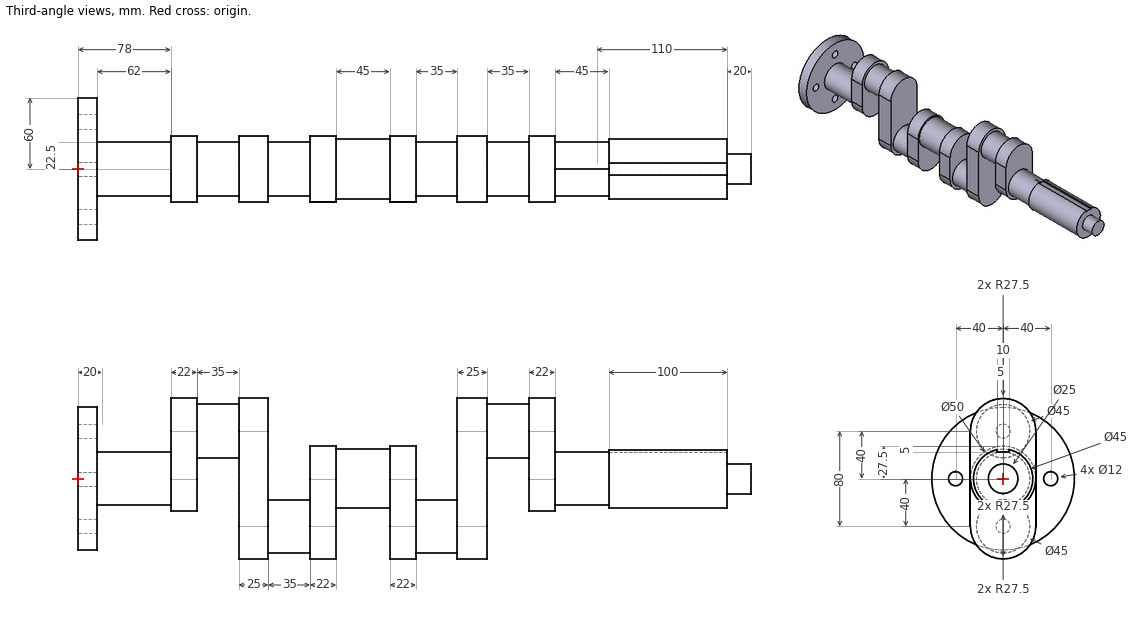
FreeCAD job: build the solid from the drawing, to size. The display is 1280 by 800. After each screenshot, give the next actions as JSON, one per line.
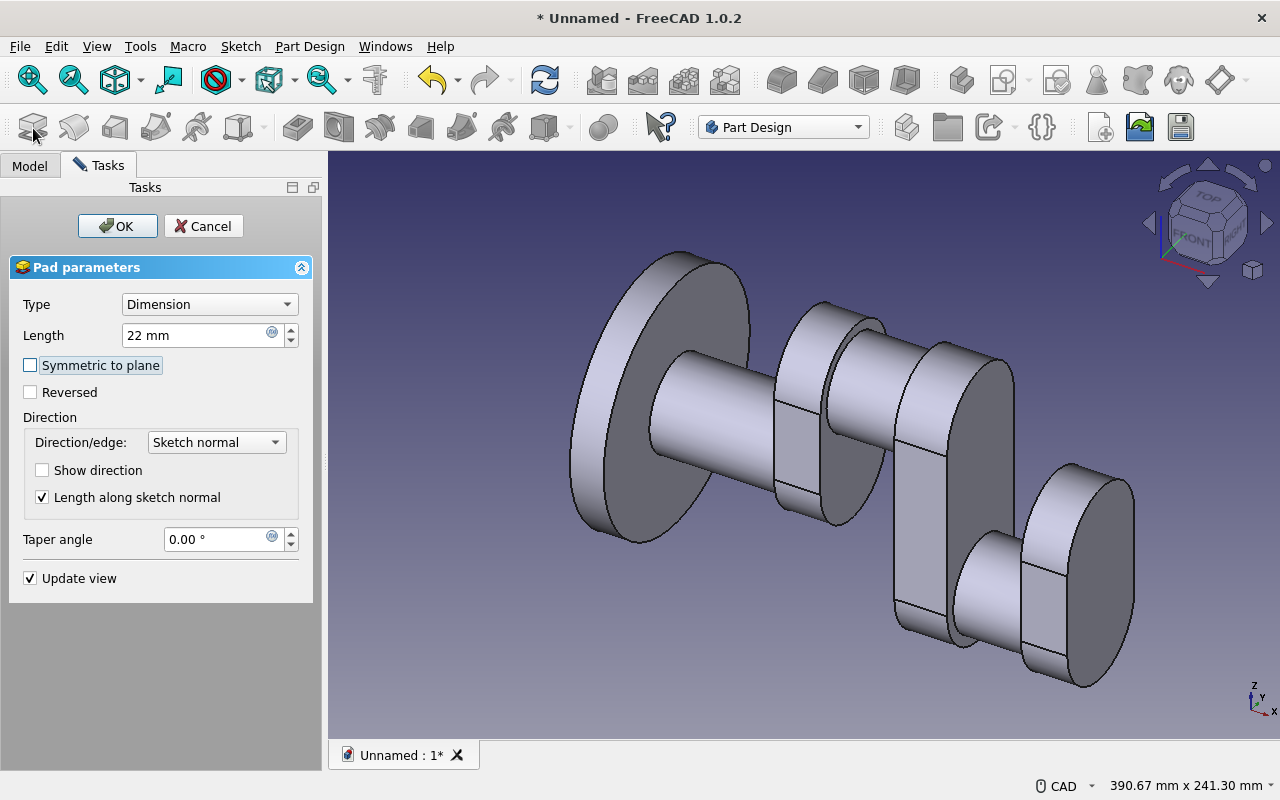
{"action": "left_click", "coordinate": [118, 226]}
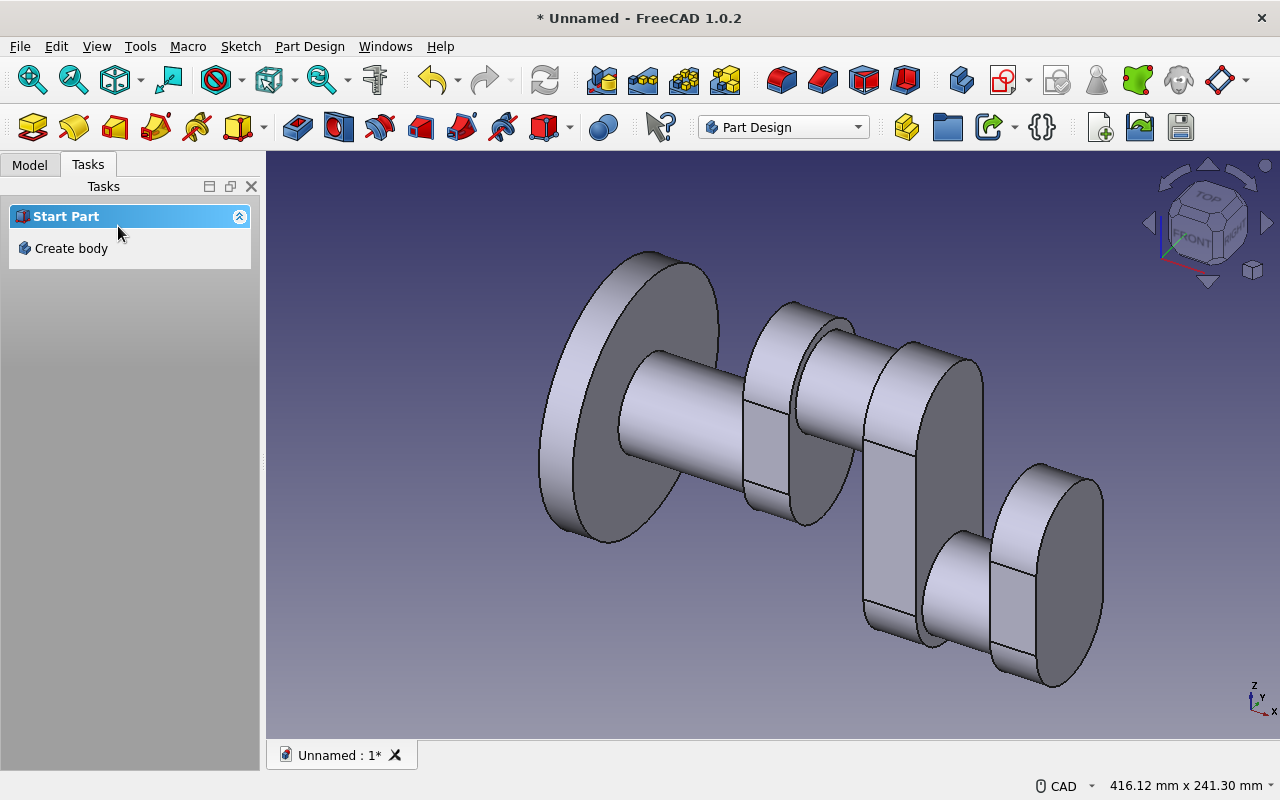
{"action": "left_click", "coordinate": [33, 80]}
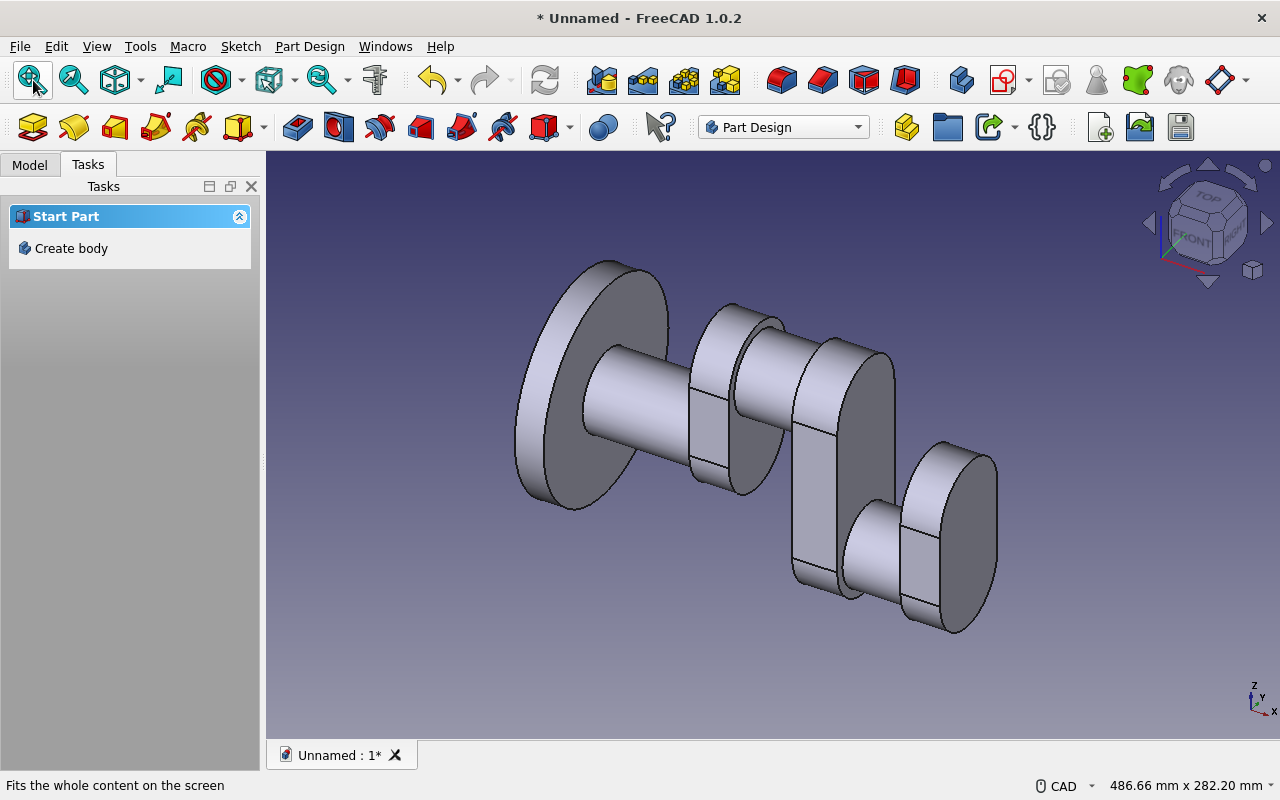
{"action": "left_click", "coordinate": [969, 520]}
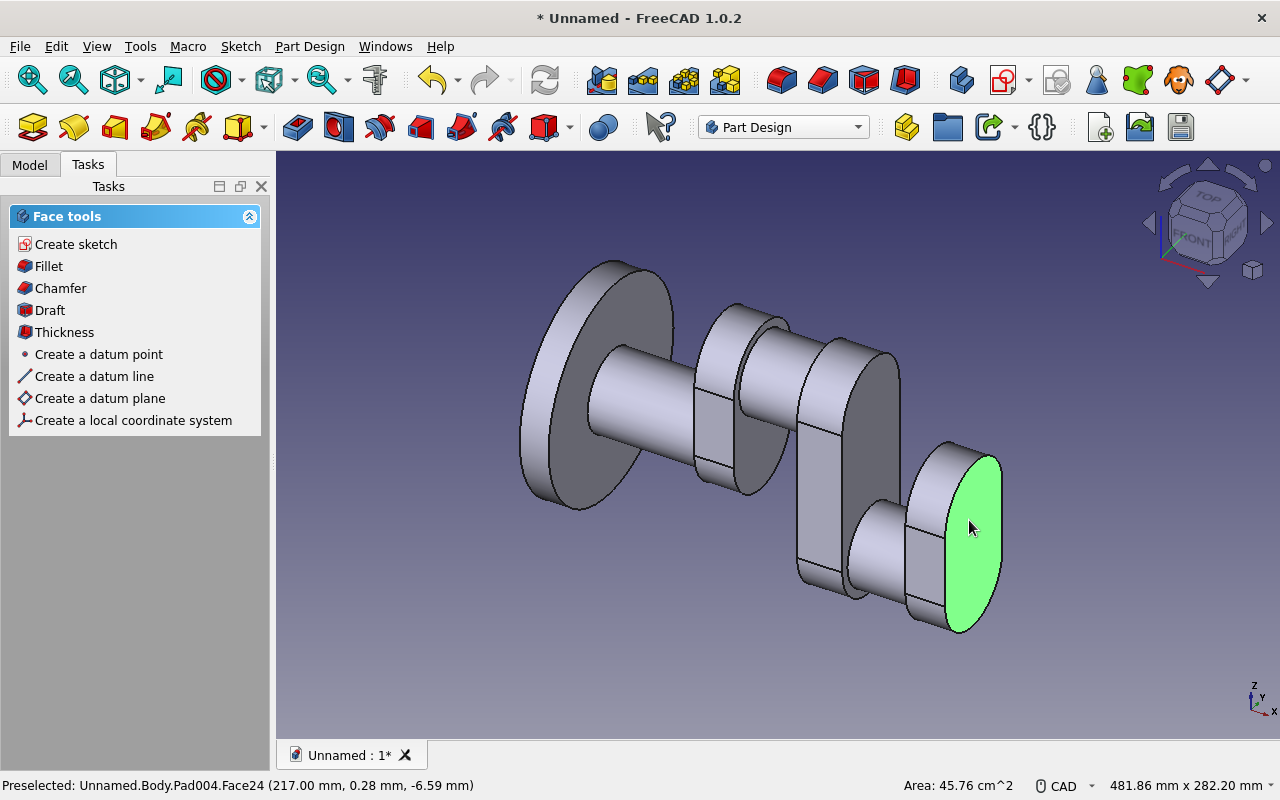
{"action": "left_click", "coordinate": [1002, 80]}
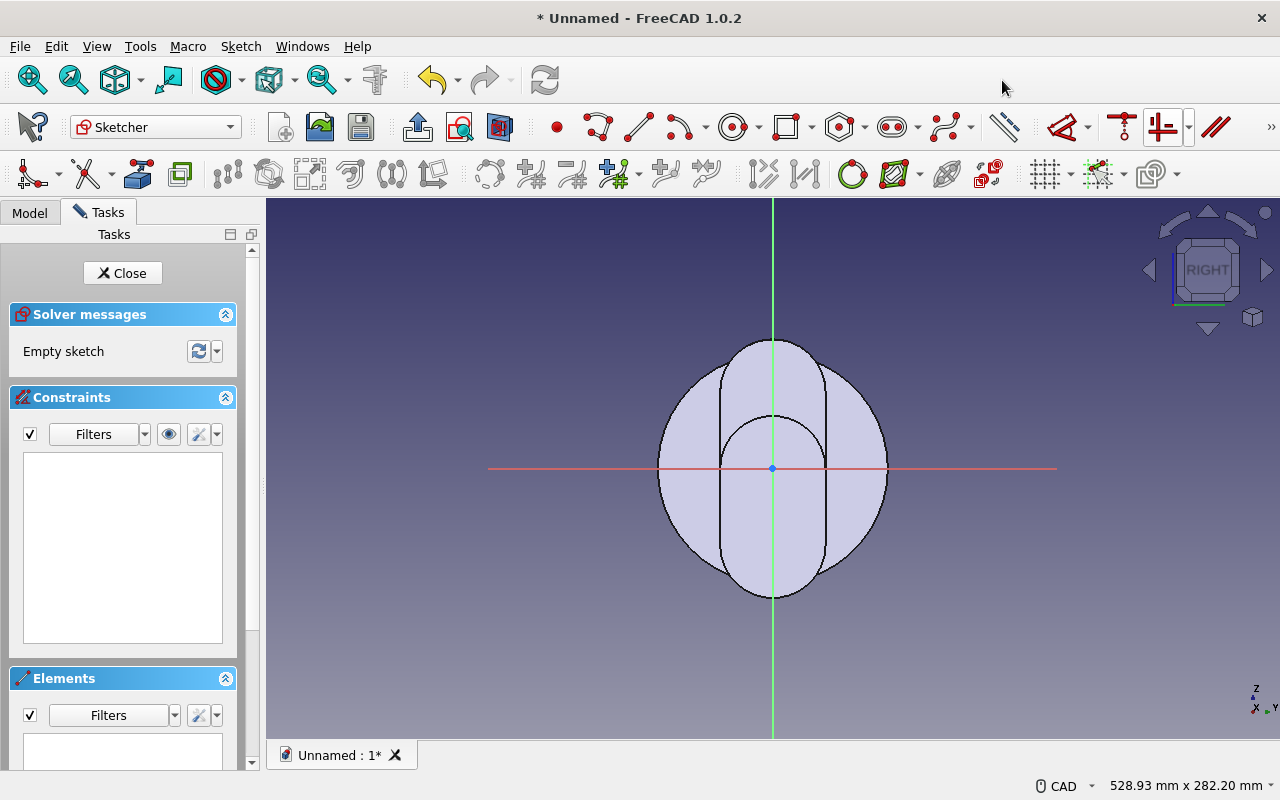
{"action": "scroll", "coordinate": [802, 469], "scroll_direction": "up", "scroll_amount": 6}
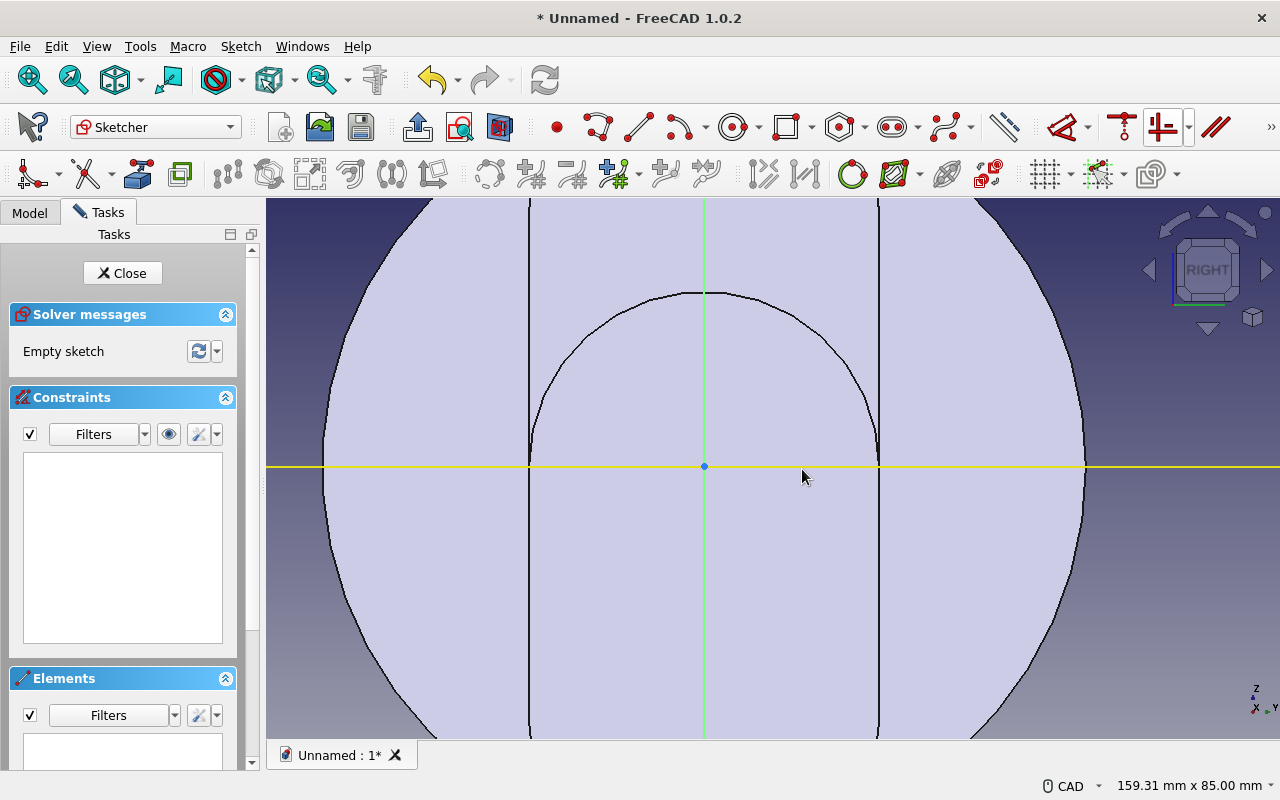
{"action": "key", "text": "g c"}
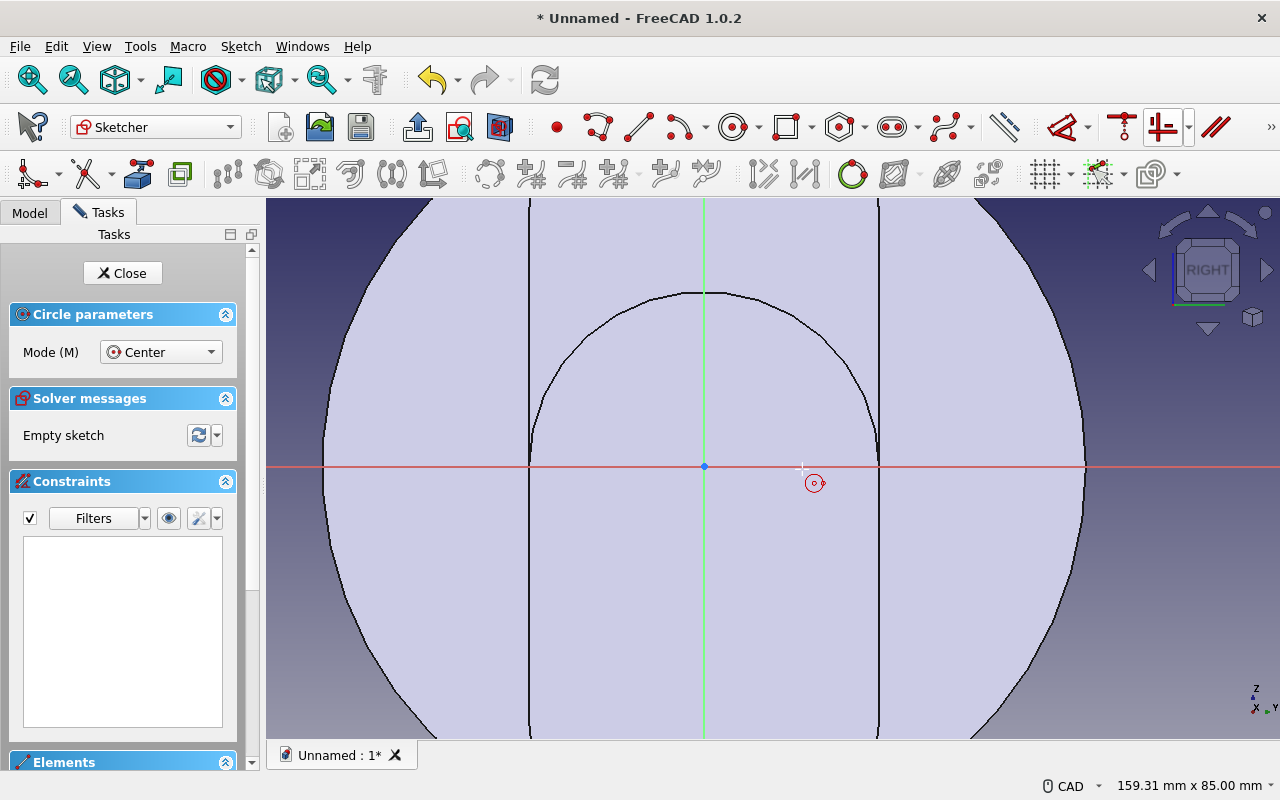
{"action": "left_click", "coordinate": [704, 467]}
{"action": "left_click", "coordinate": [817, 354]}
{"action": "key", "text": "Escape"}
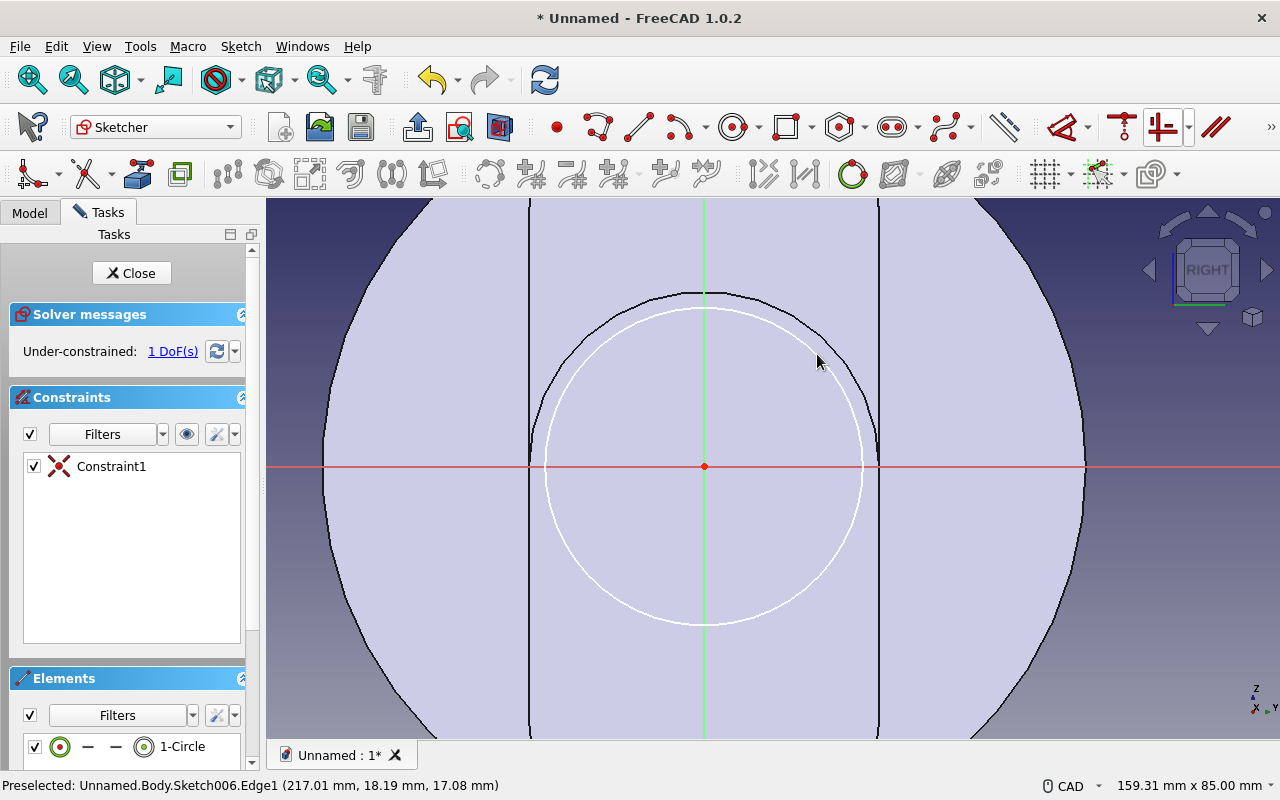
{"action": "left_click", "coordinate": [1062, 128]}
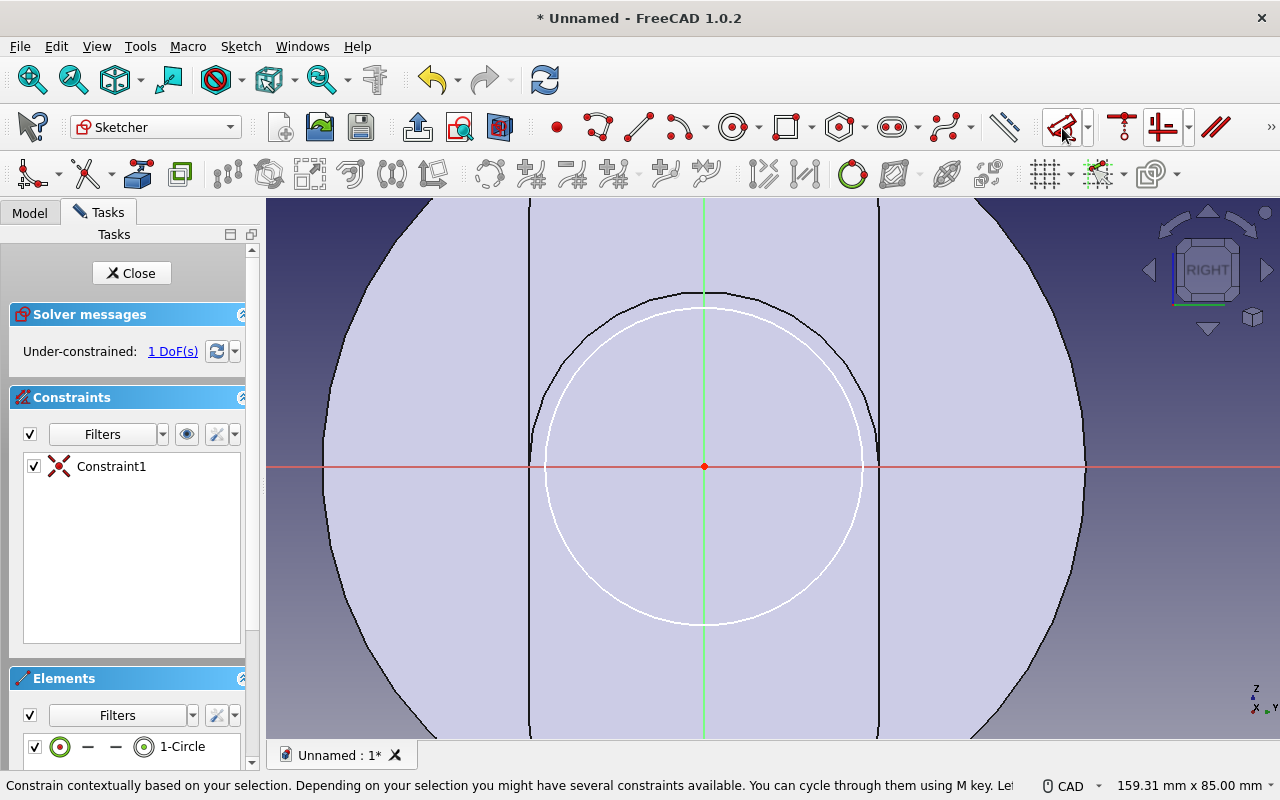
{"action": "left_click", "coordinate": [816, 354]}
{"action": "left_click", "coordinate": [839, 331]}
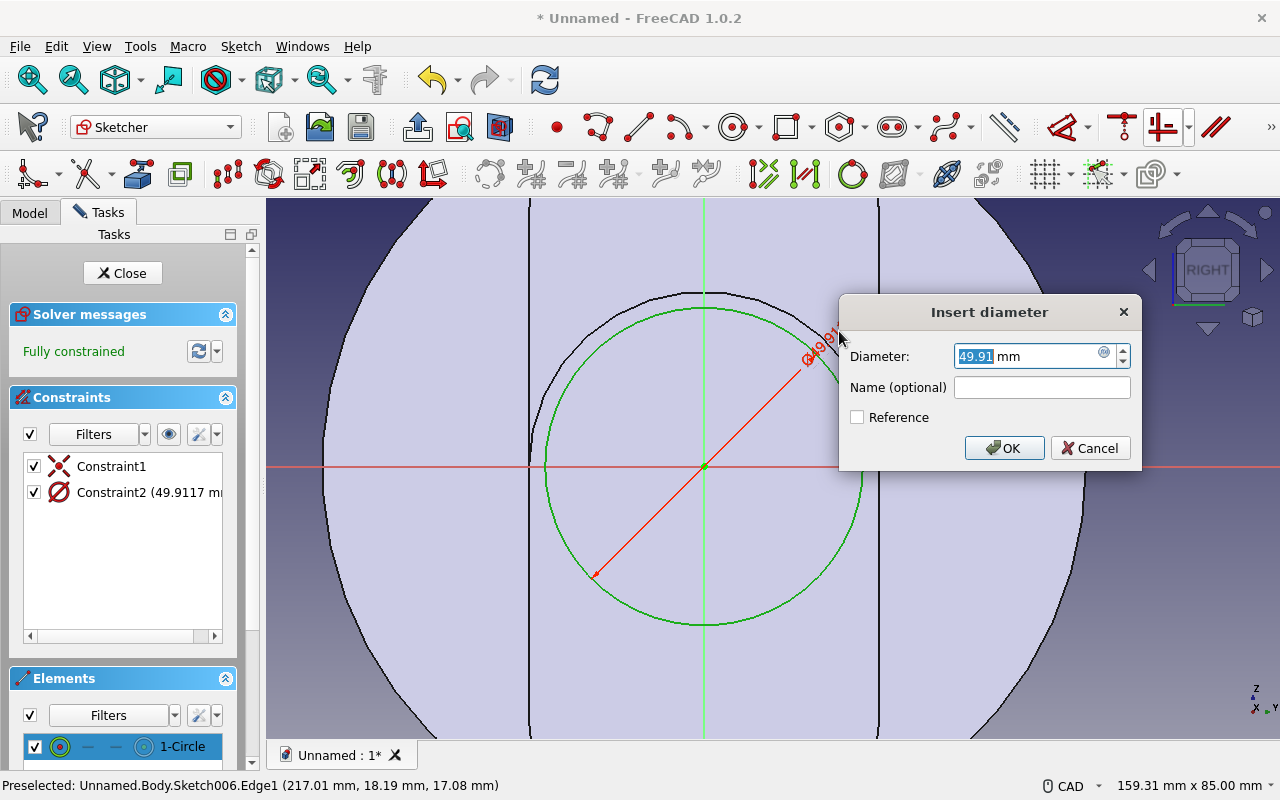
{"action": "type", "text": "50"}
{"action": "key", "text": "Return"}
{"action": "key", "text": "Escape"}